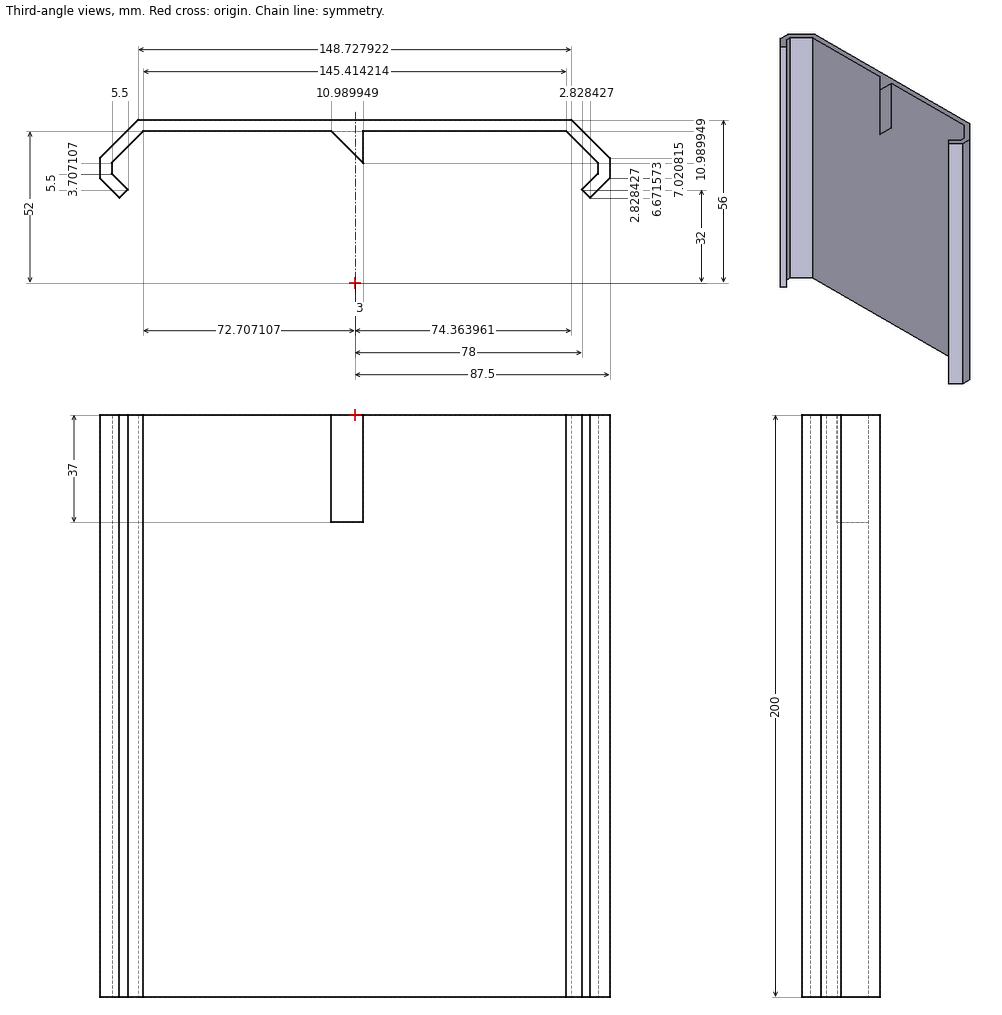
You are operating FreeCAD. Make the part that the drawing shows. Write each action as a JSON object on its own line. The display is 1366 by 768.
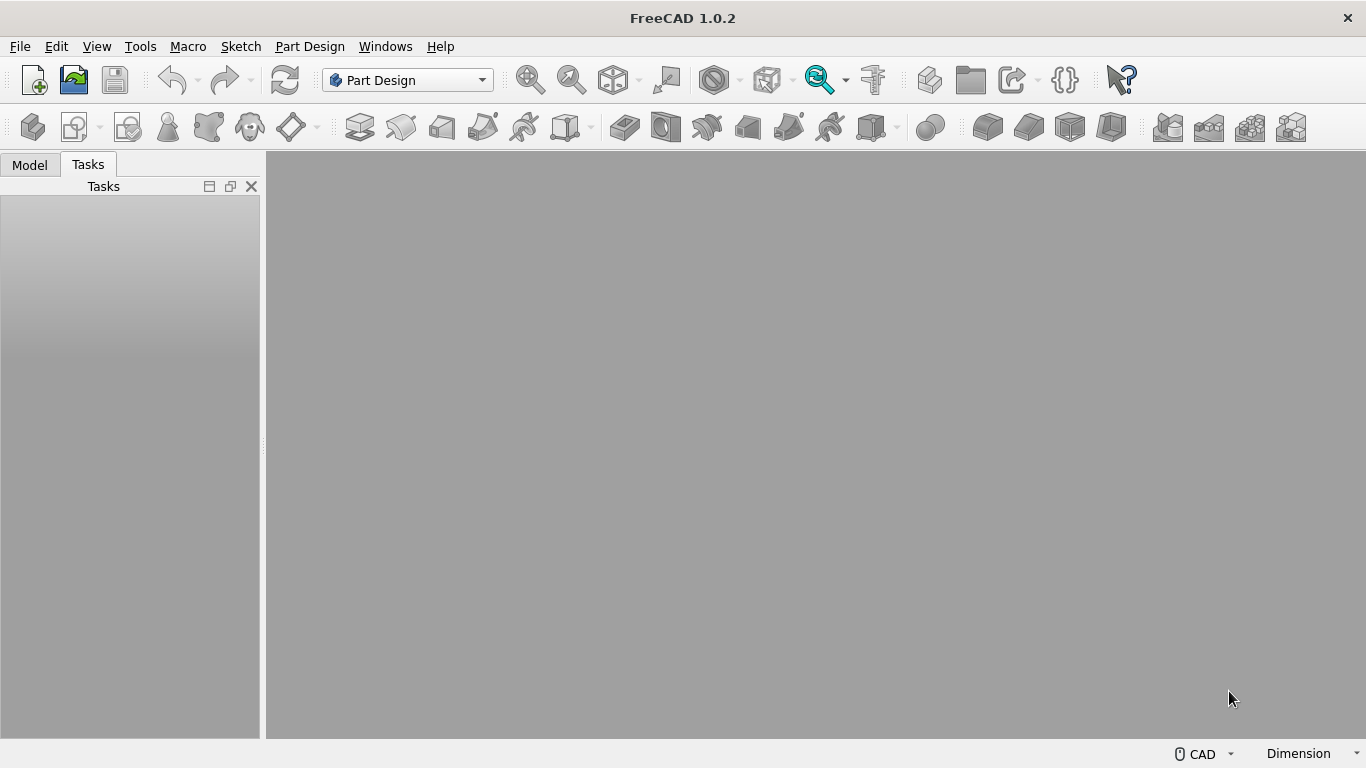
{"action": "left_click", "coordinate": [33, 80]}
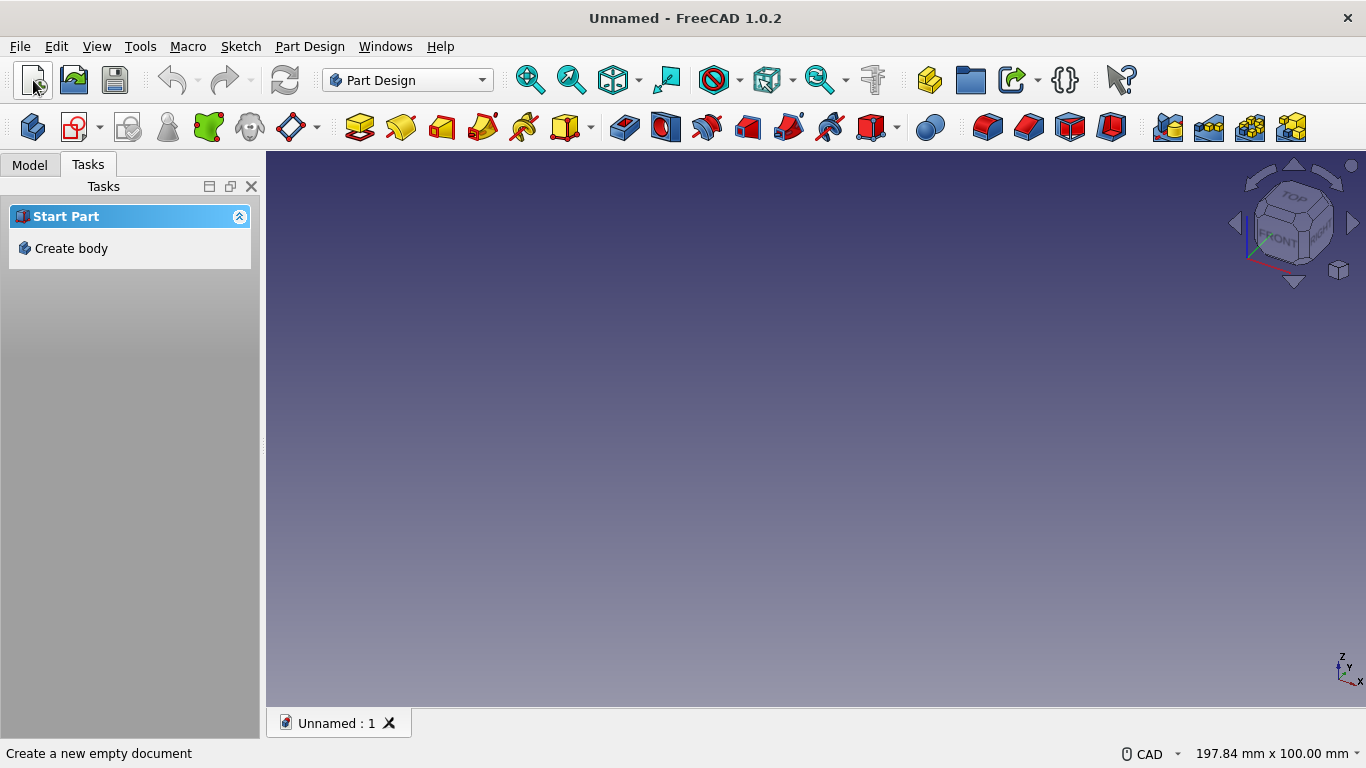
{"action": "left_click", "coordinate": [74, 128]}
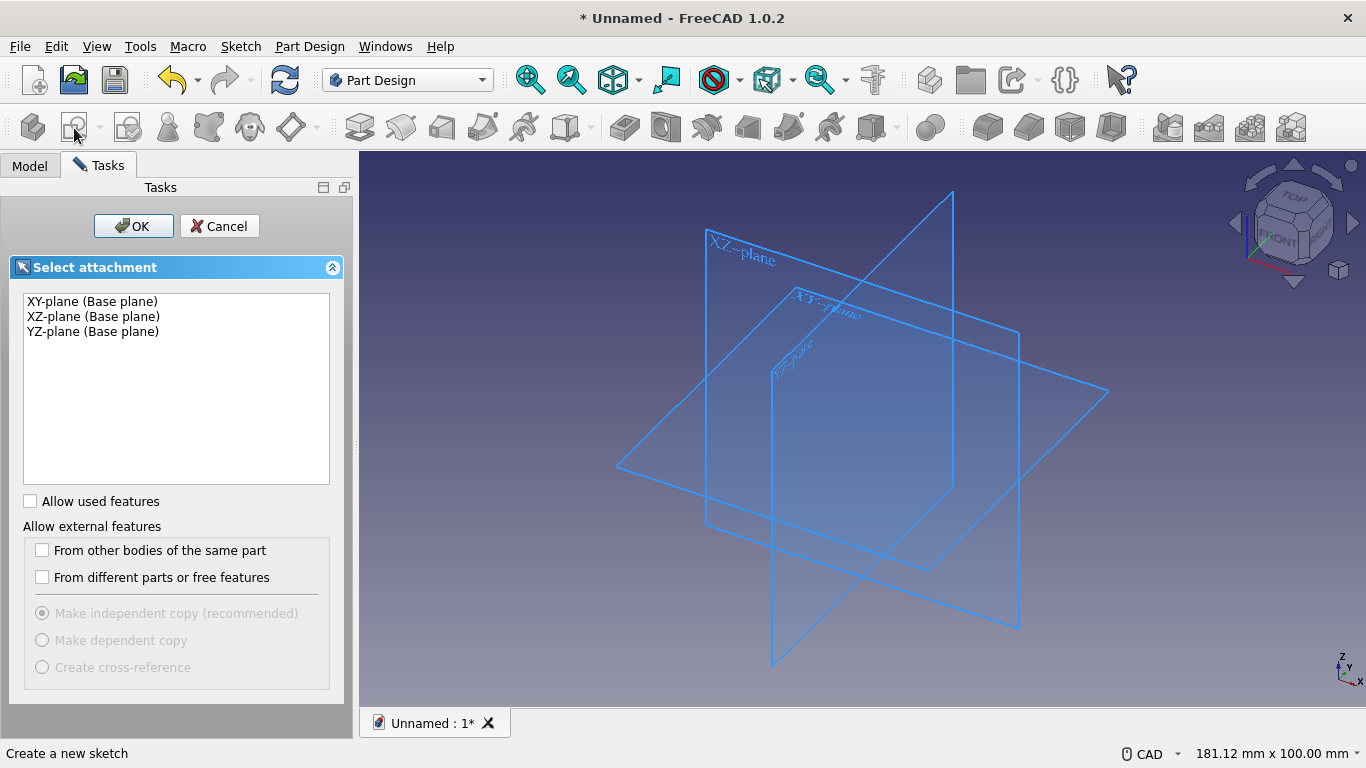
{"action": "left_click", "coordinate": [84, 302]}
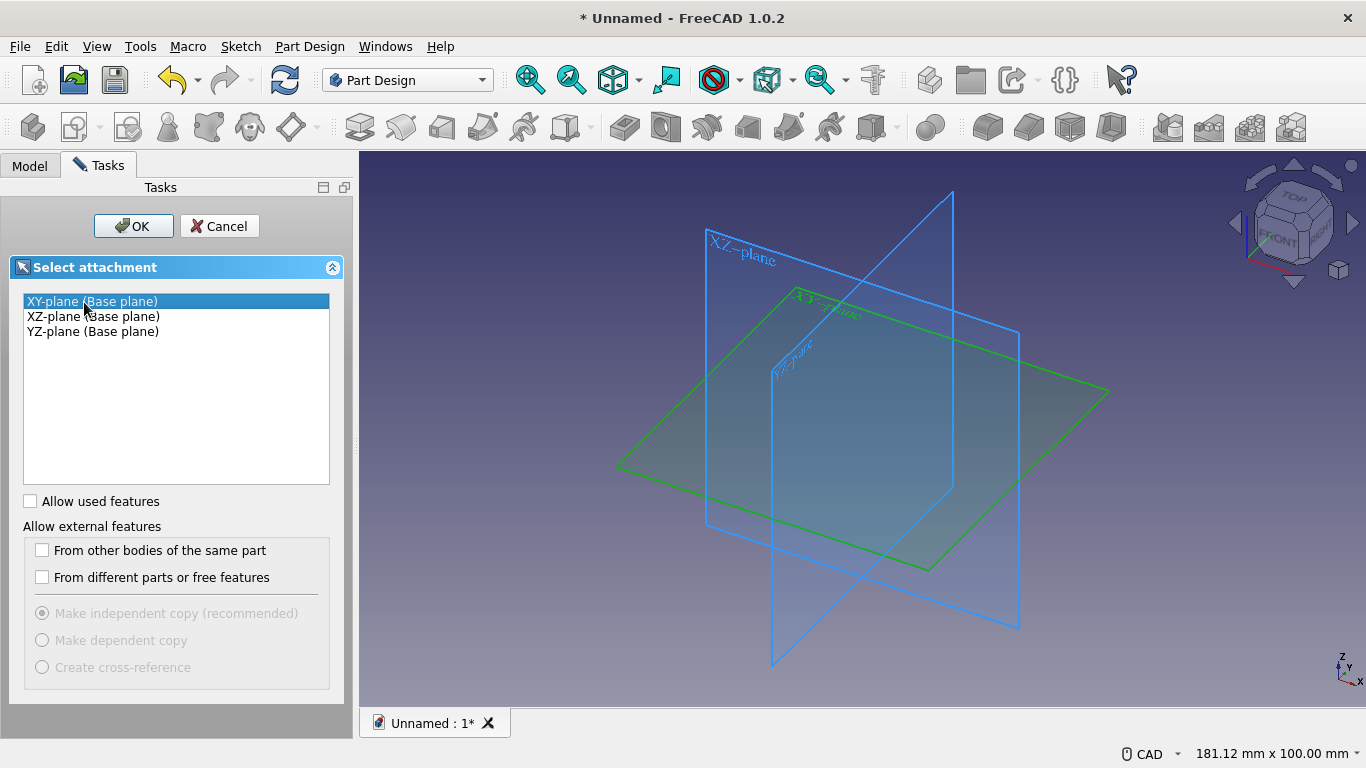
{"action": "left_click", "coordinate": [134, 226]}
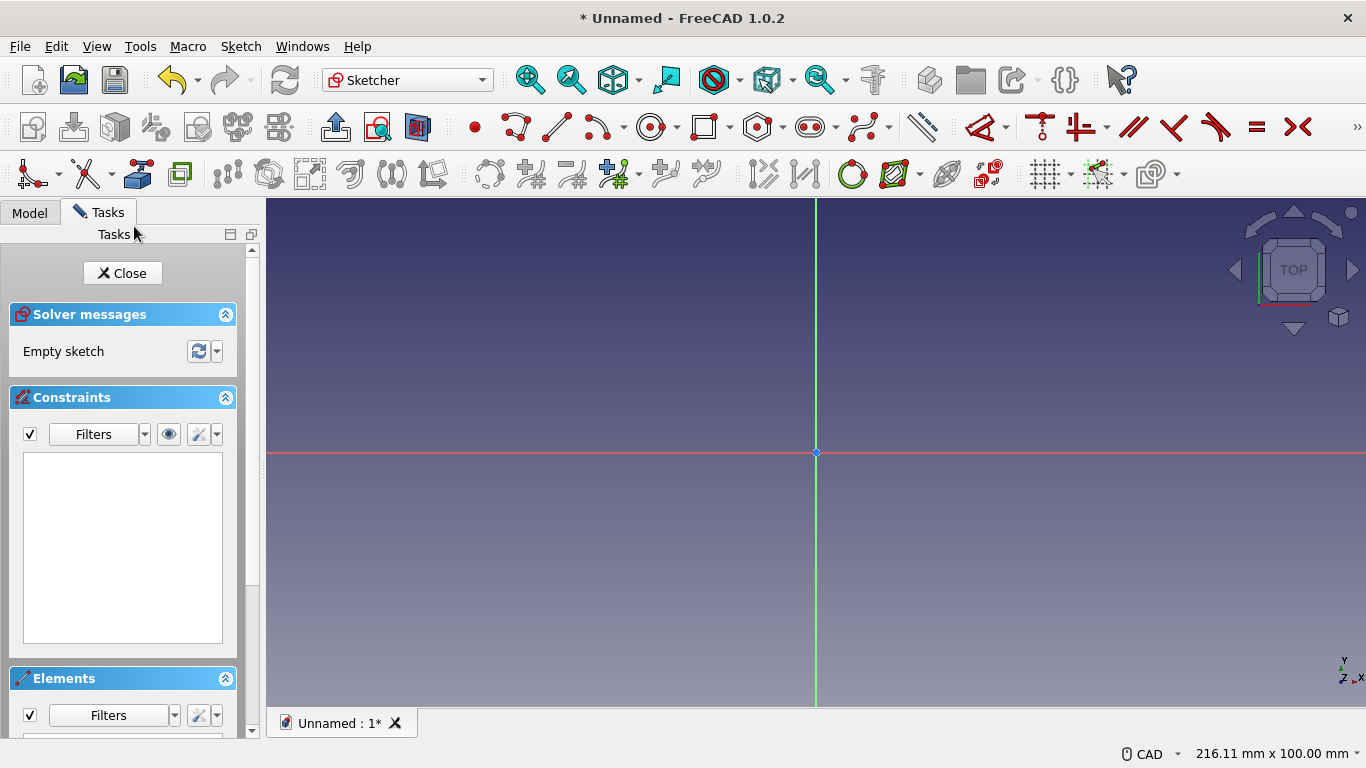
{"action": "scroll", "coordinate": [608, 679], "scroll_direction": "down", "scroll_amount": 2}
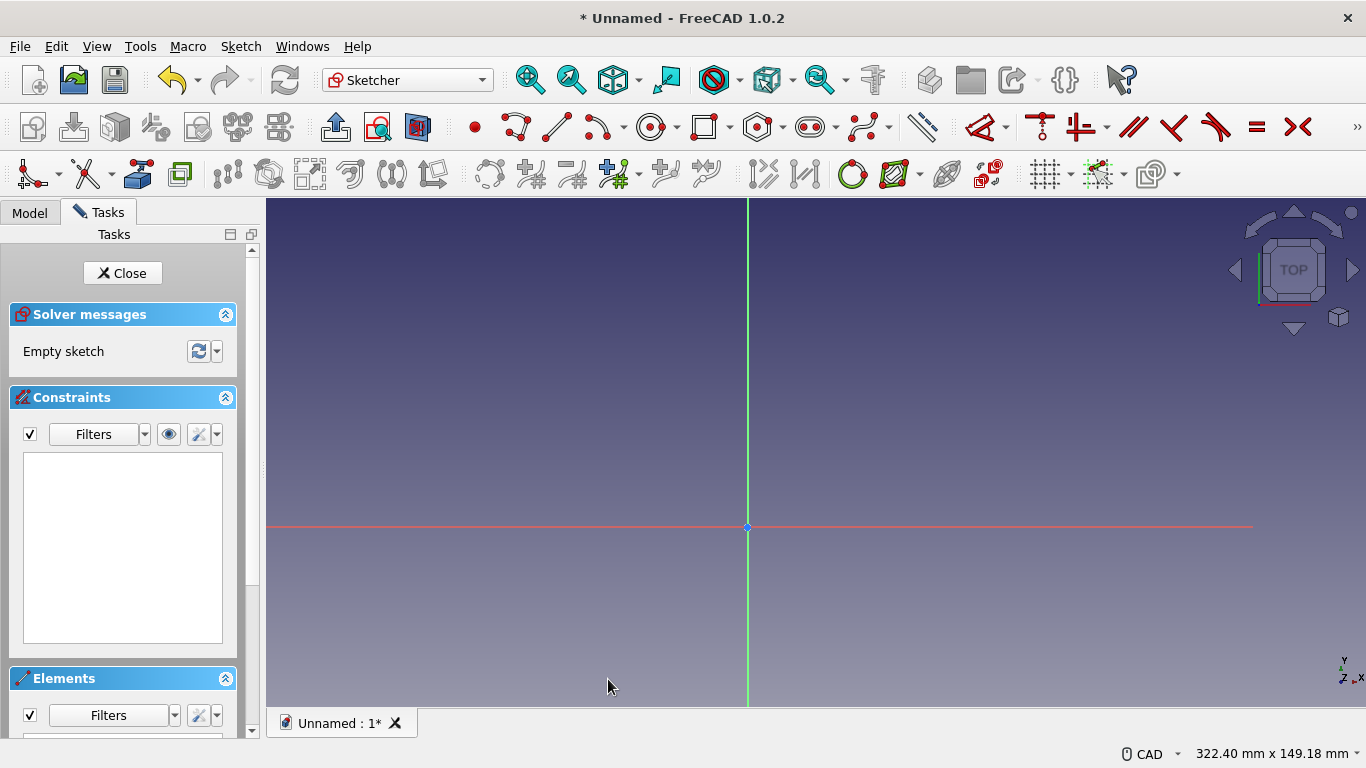
{"action": "left_click", "coordinate": [516, 128]}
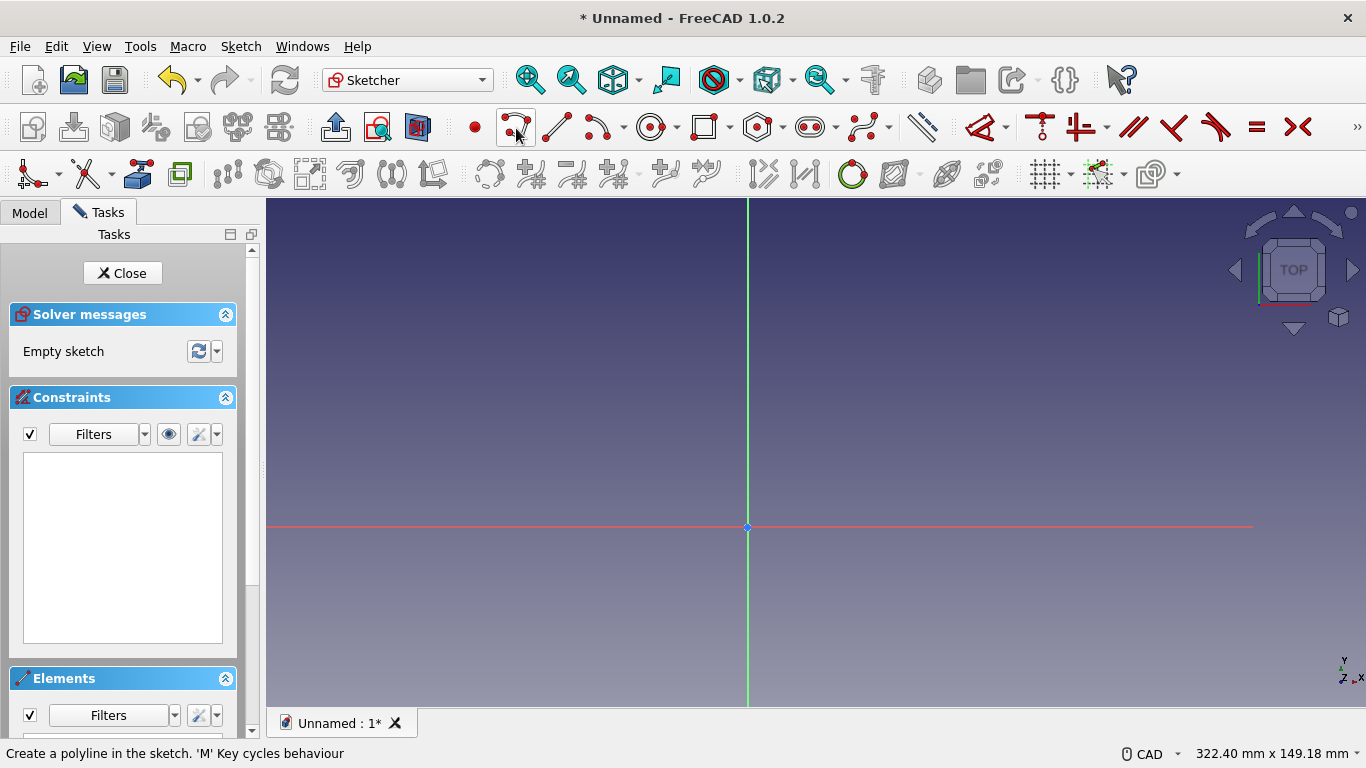
{"action": "left_click", "coordinate": [1014, 418]}
{"action": "left_click", "coordinate": [1023, 428]}
{"action": "left_click", "coordinate": [1046, 405]}
{"action": "left_click", "coordinate": [1046, 381]}
{"action": "left_click", "coordinate": [1001, 336]}
{"action": "left_click", "coordinate": [494, 336]}
{"action": "left_click", "coordinate": [449, 381]}
{"action": "left_click", "coordinate": [449, 405]}
{"action": "left_click", "coordinate": [472, 428]}
{"action": "left_click", "coordinate": [481, 418]}
{"action": "left_click", "coordinate": [463, 400]}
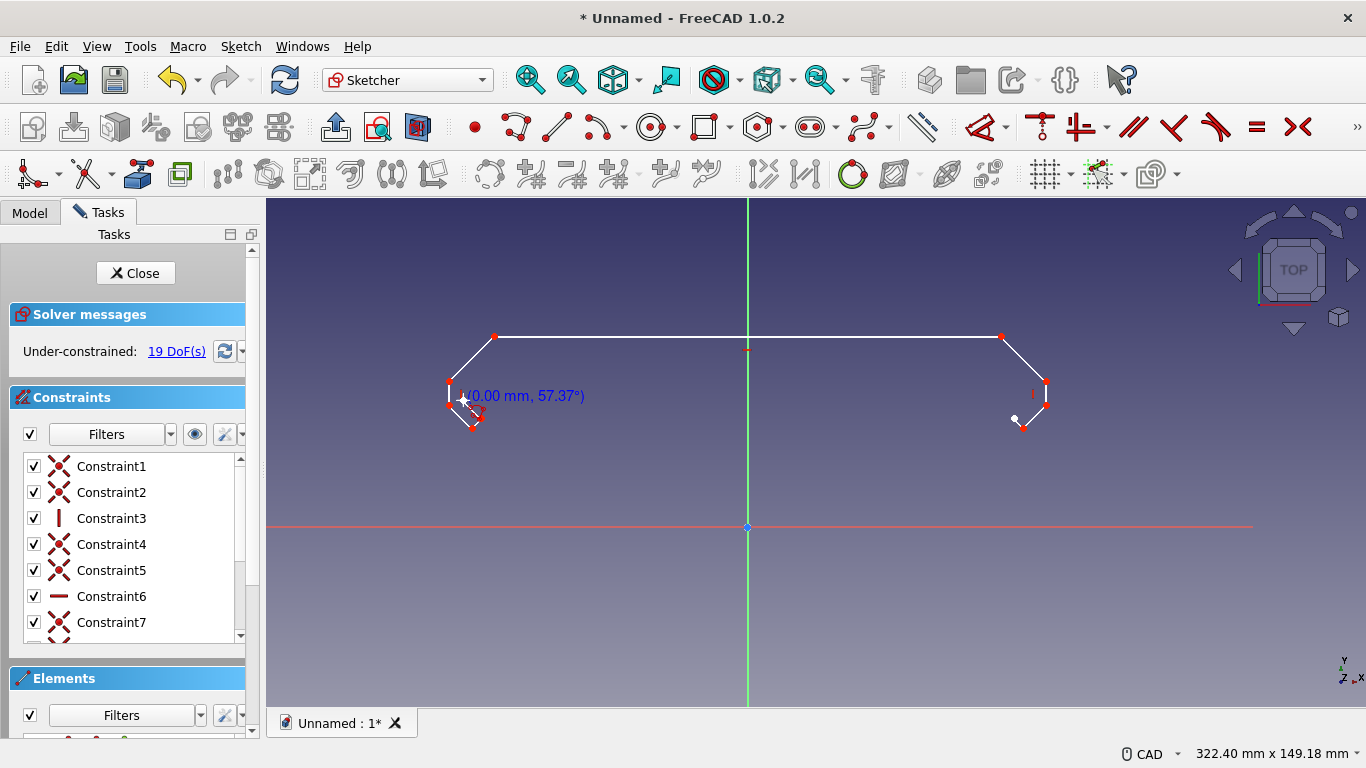
{"action": "scroll", "coordinate": [463, 387], "scroll_direction": "up", "scroll_amount": 2}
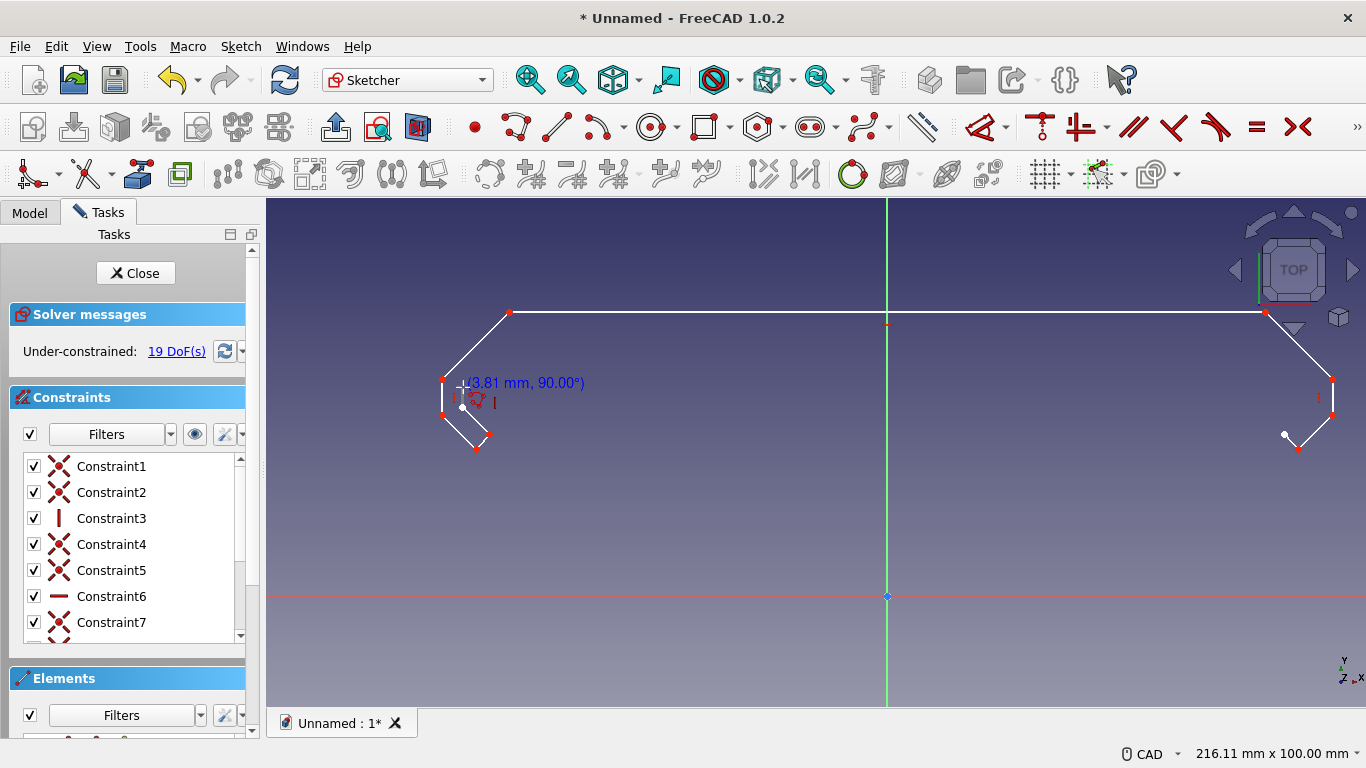
{"action": "left_click", "coordinate": [463, 387]}
{"action": "left_click", "coordinate": [517, 332]}